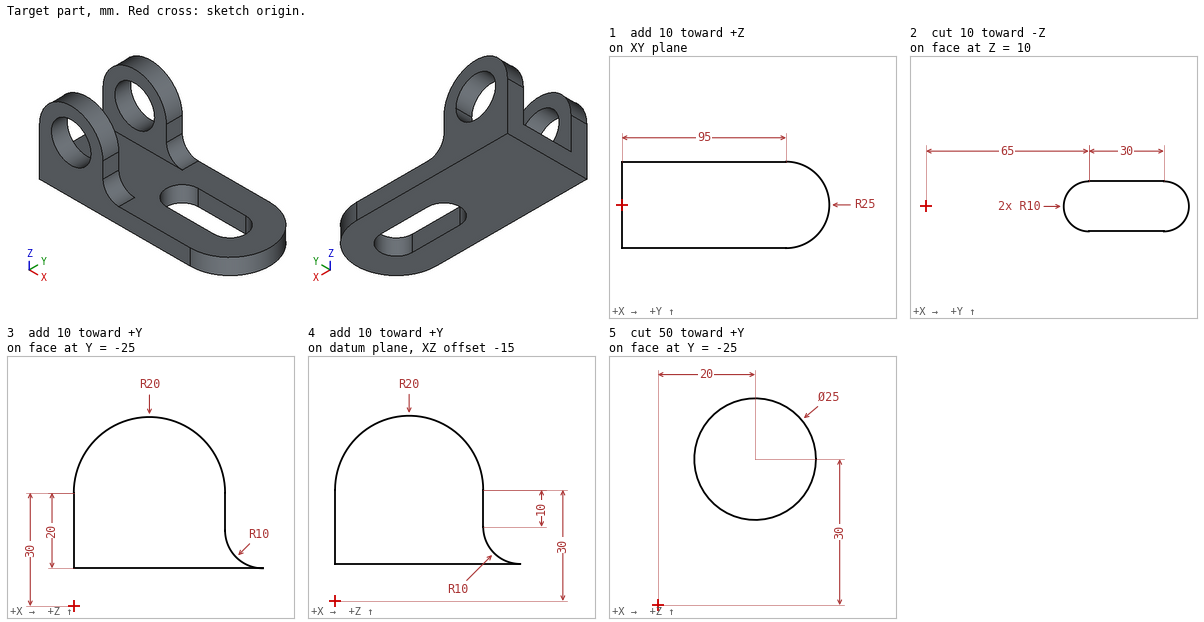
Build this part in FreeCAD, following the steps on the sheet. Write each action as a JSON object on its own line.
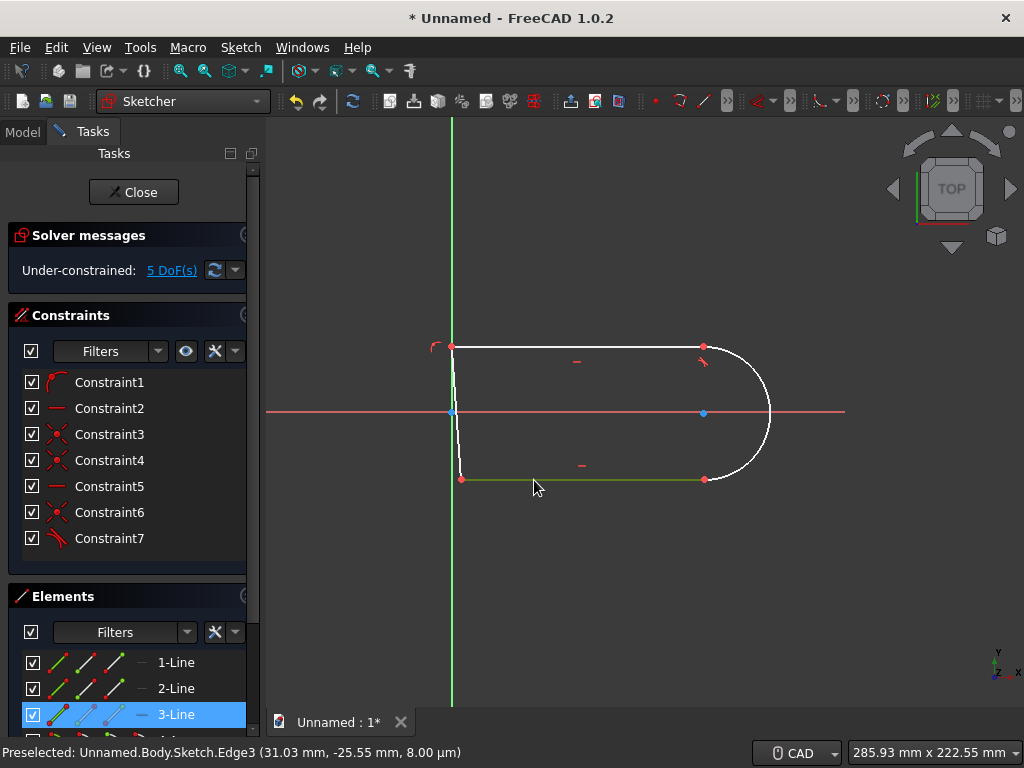
{"action": "left_click", "coordinate": [758, 452]}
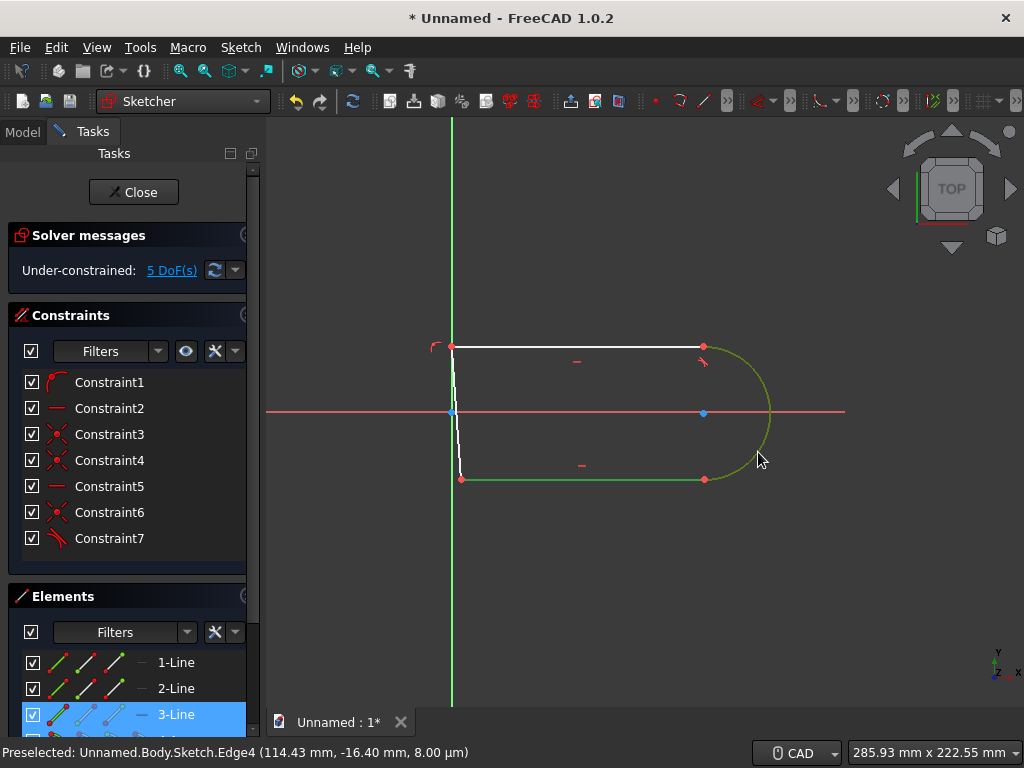
{"action": "key", "text": "t"}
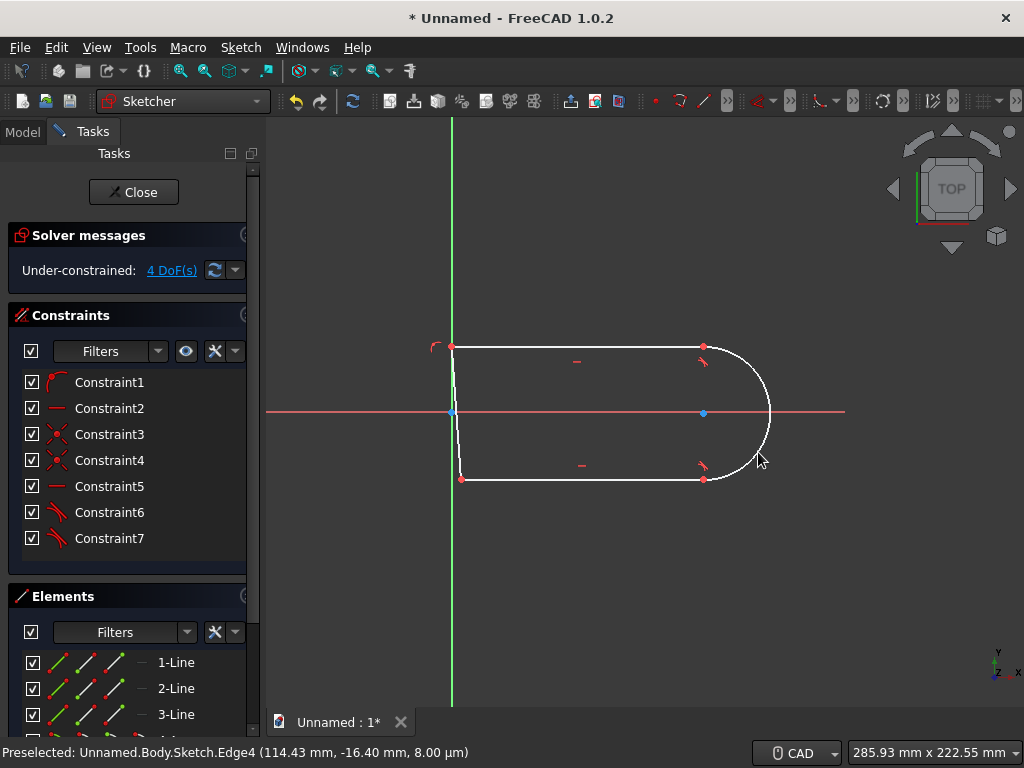
{"action": "left_click", "coordinate": [455, 387]}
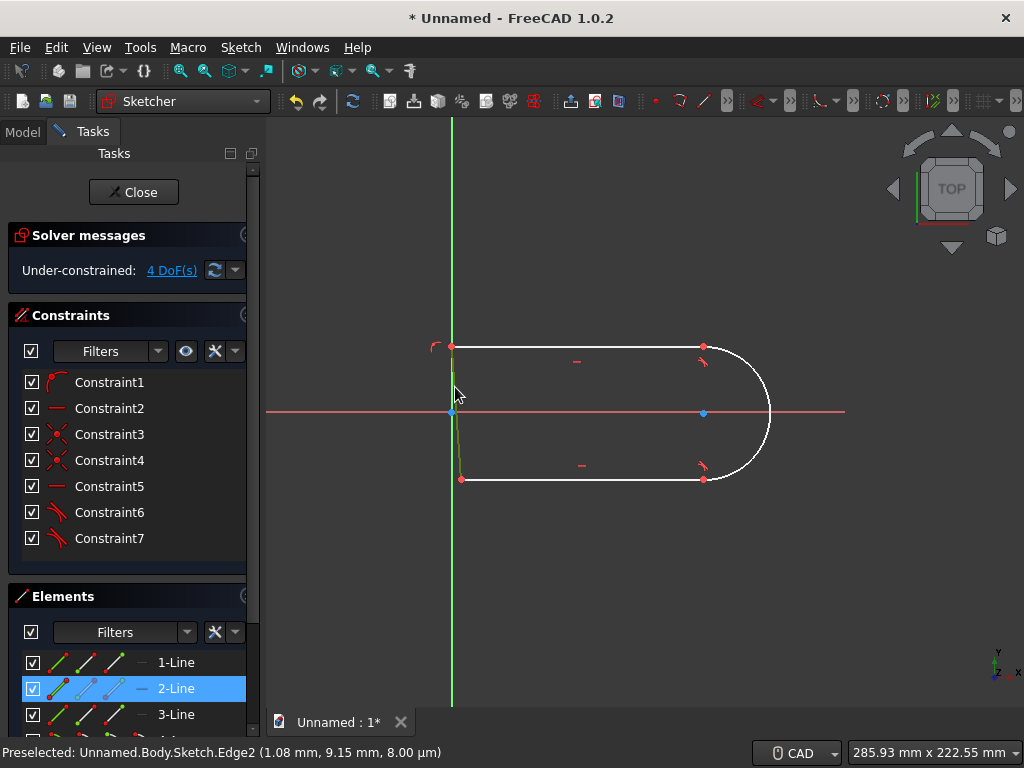
{"action": "key", "text": "v"}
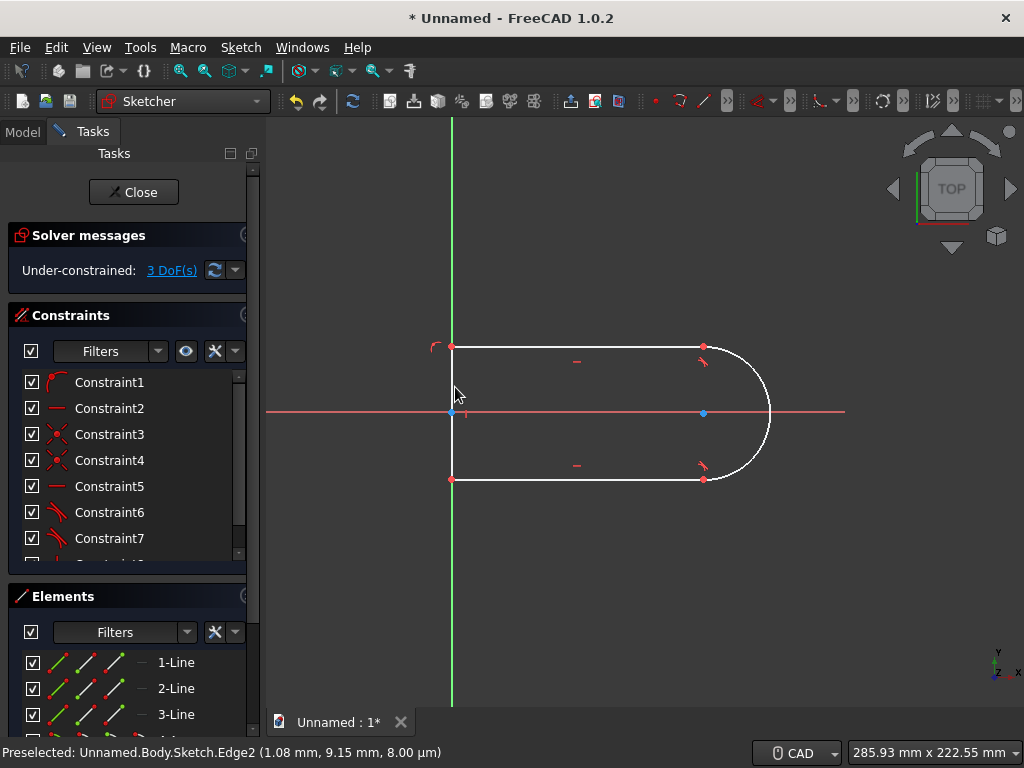
{"action": "left_click", "coordinate": [704, 414]}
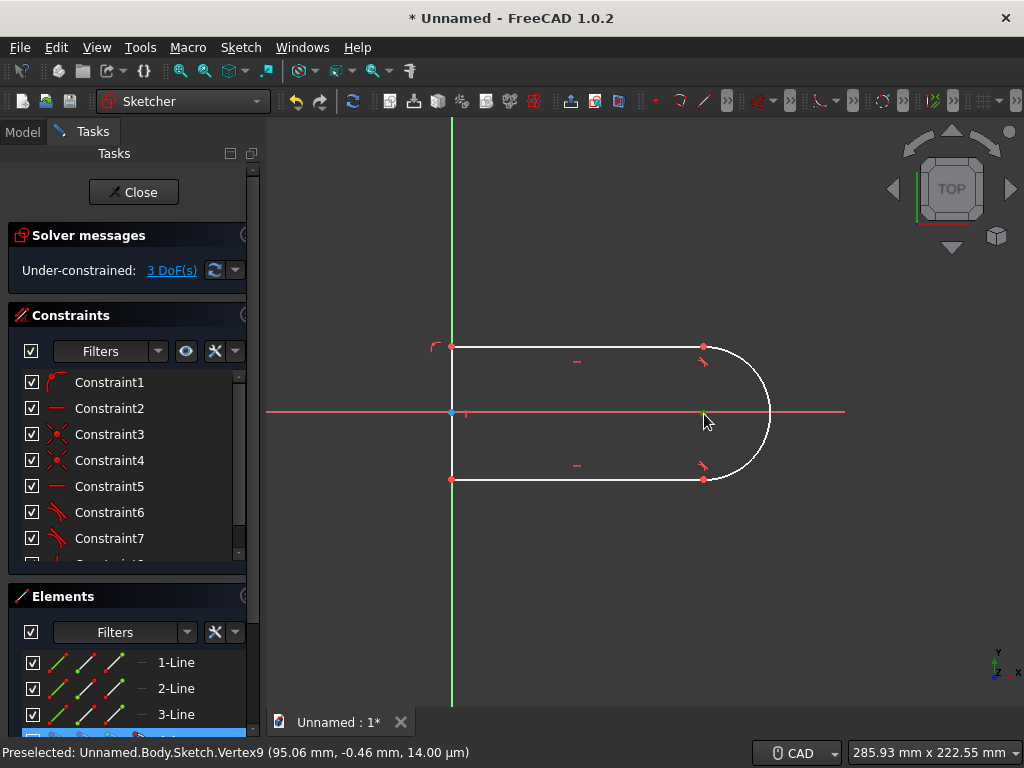
{"action": "left_click", "coordinate": [334, 412]}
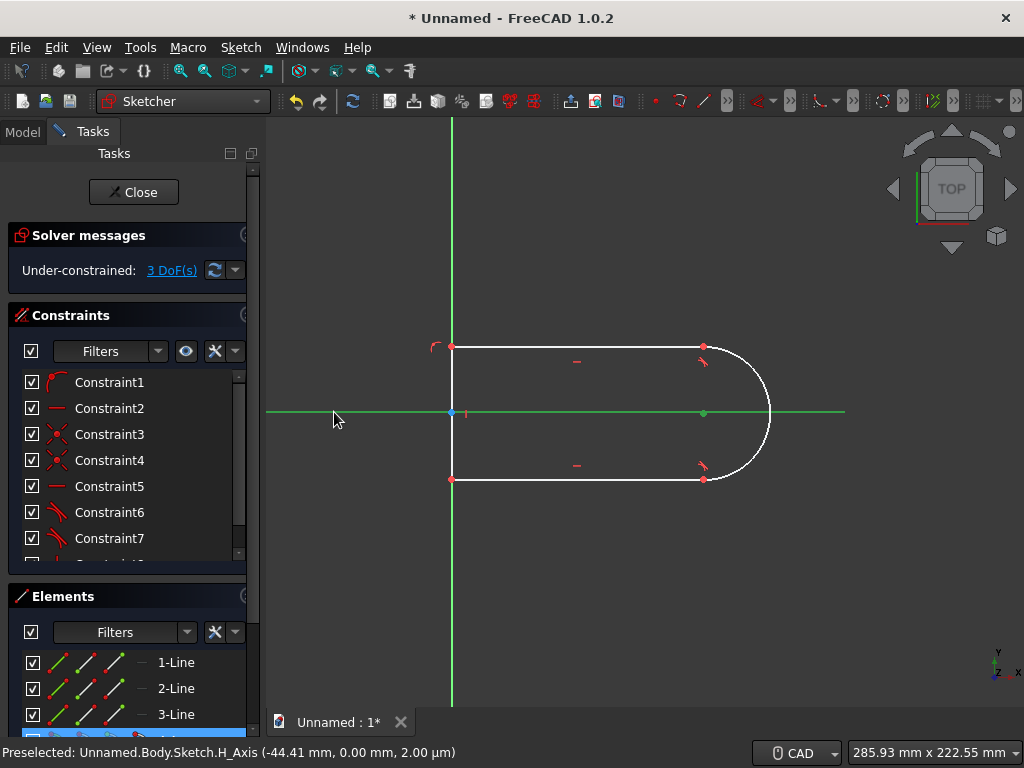
{"action": "key", "text": "c"}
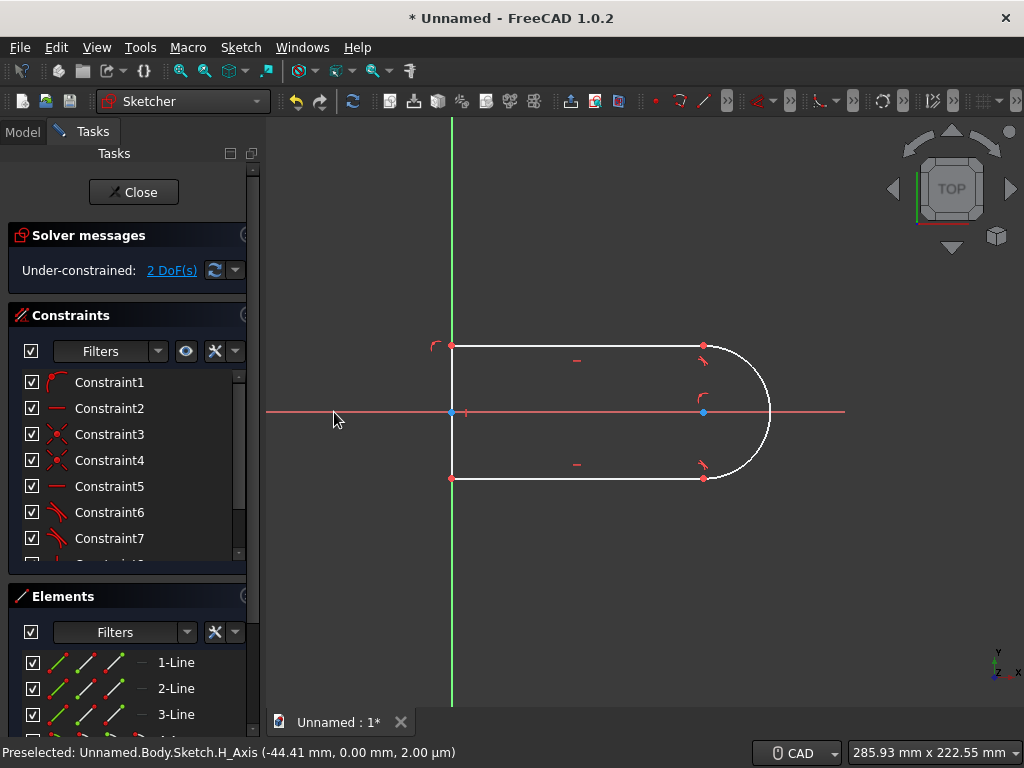
{"action": "left_click", "coordinate": [758, 451]}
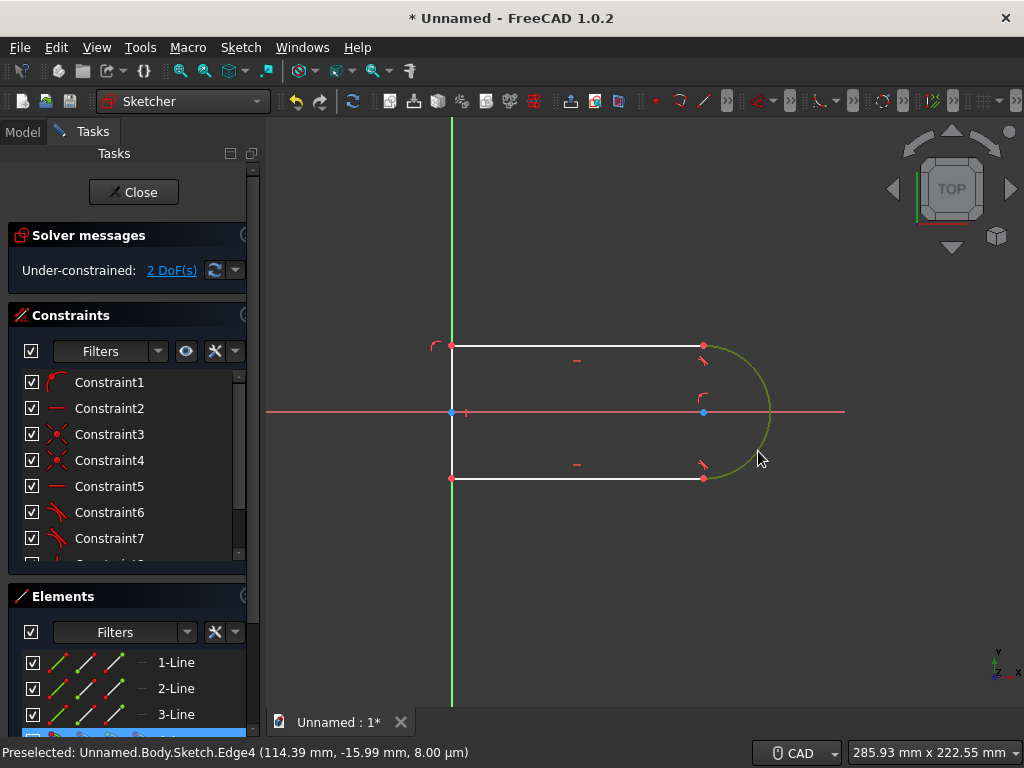
{"action": "key", "text": "k r"}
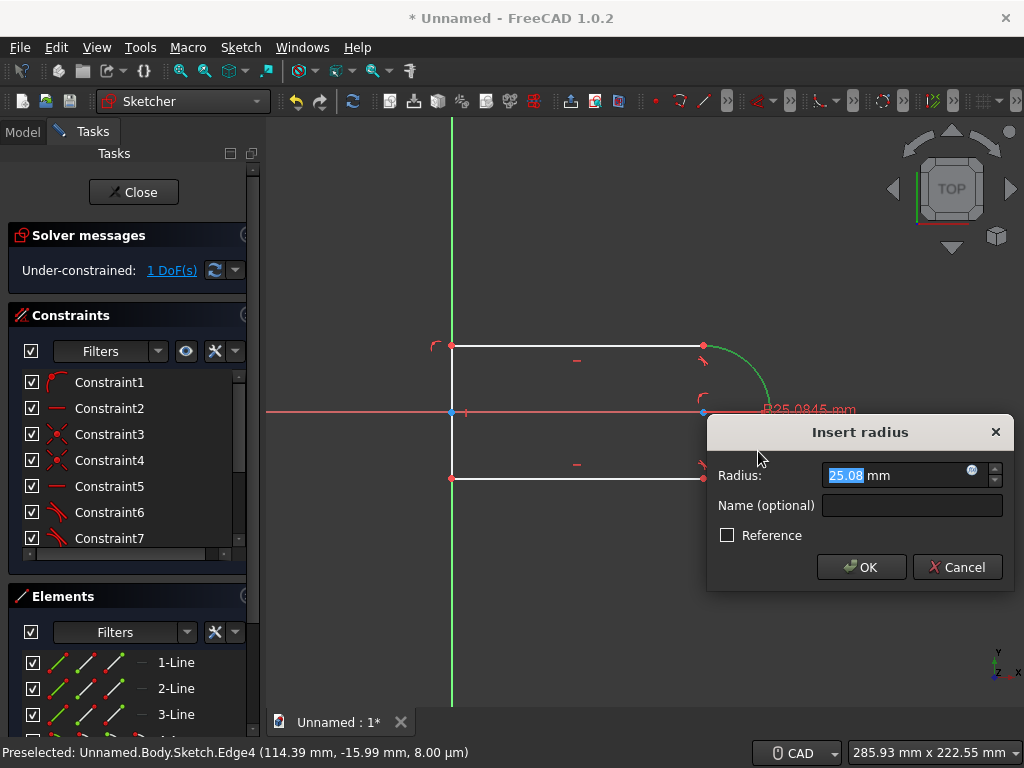
{"action": "type", "text": "25"}
{"action": "key", "text": "Return"}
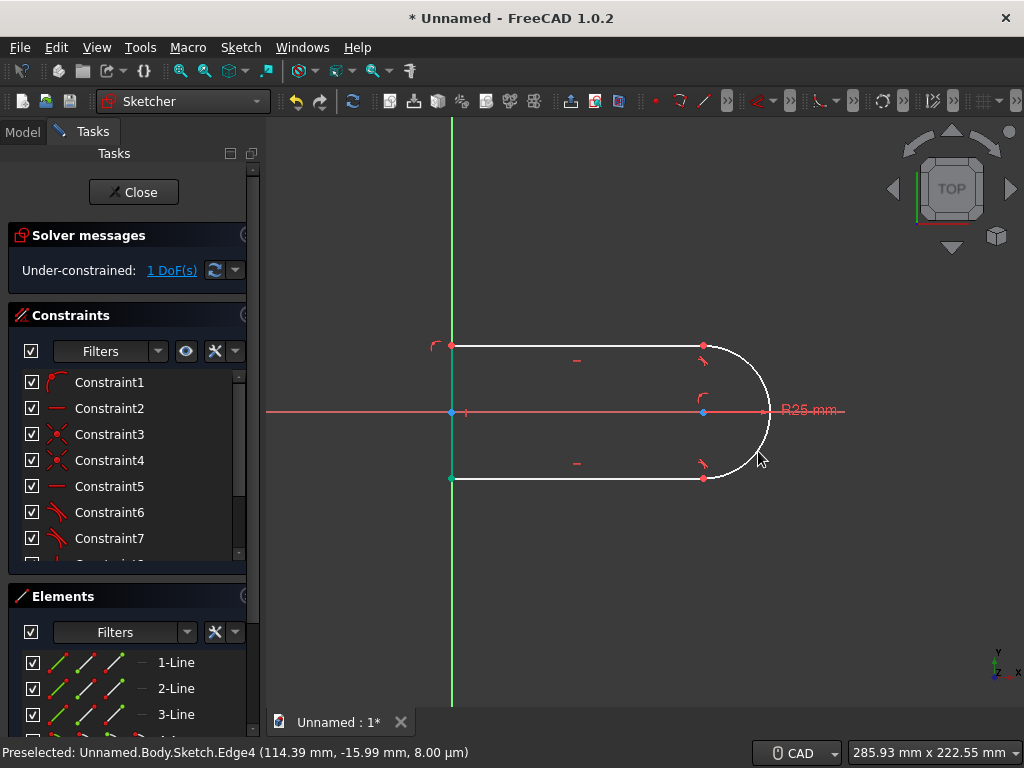
{"action": "left_click", "coordinate": [628, 346]}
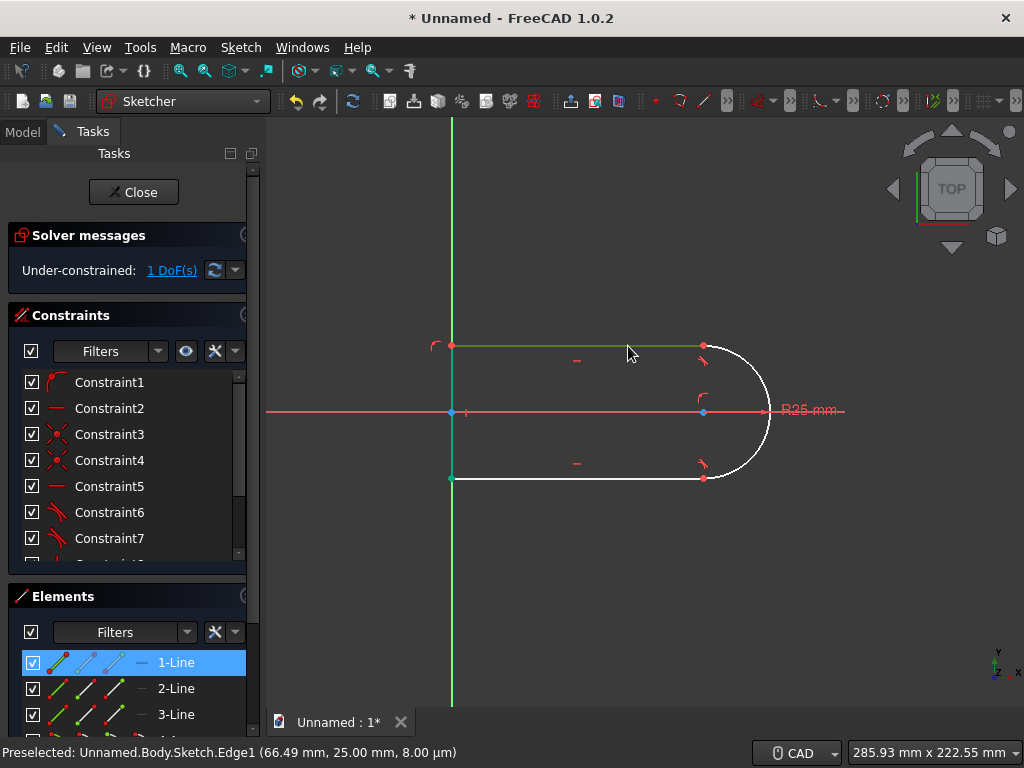
{"action": "left_click", "coordinate": [776, 102]}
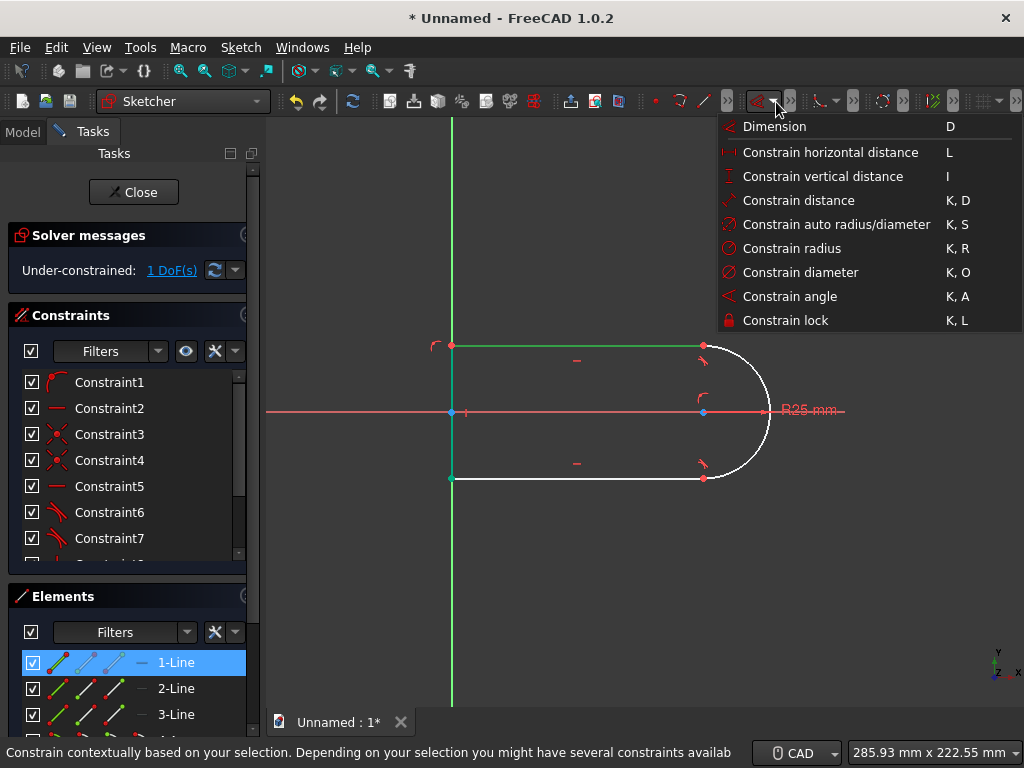
{"action": "left_click", "coordinate": [870, 152]}